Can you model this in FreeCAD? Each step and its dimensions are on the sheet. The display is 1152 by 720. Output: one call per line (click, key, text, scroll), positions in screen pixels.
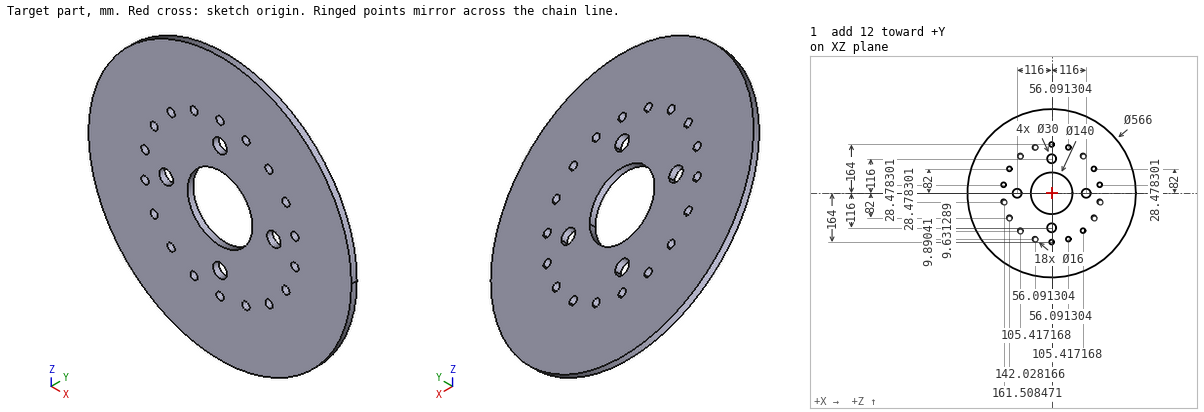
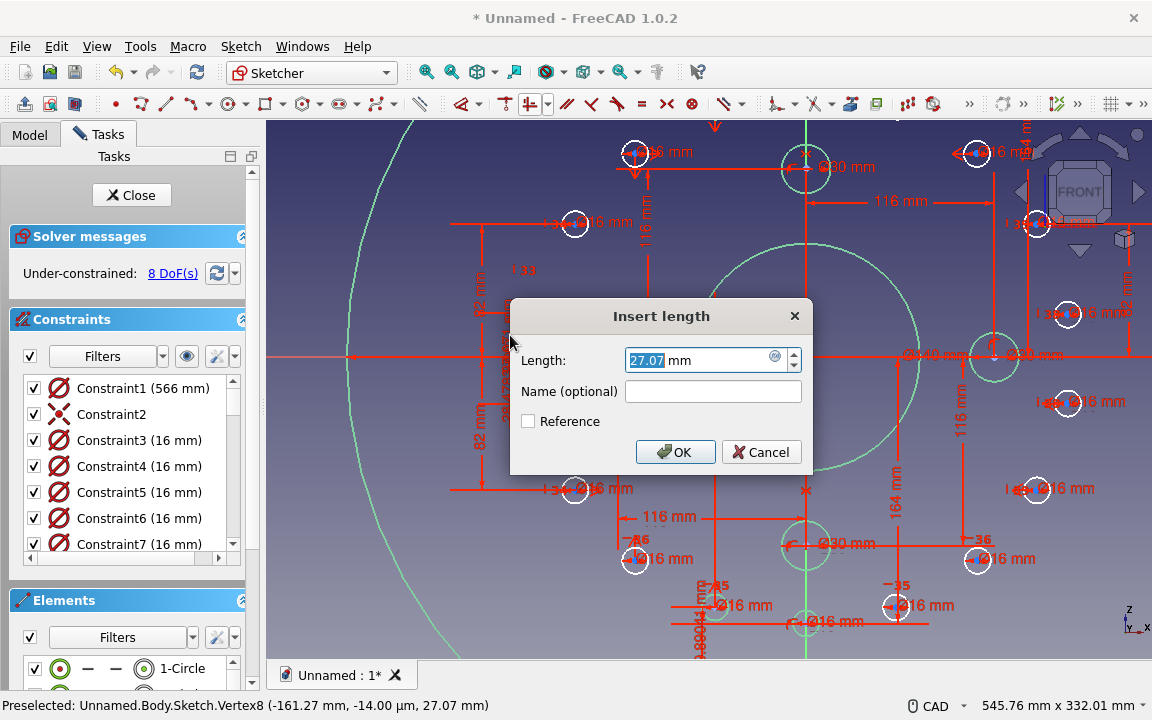
text(28.478301)
key(Return)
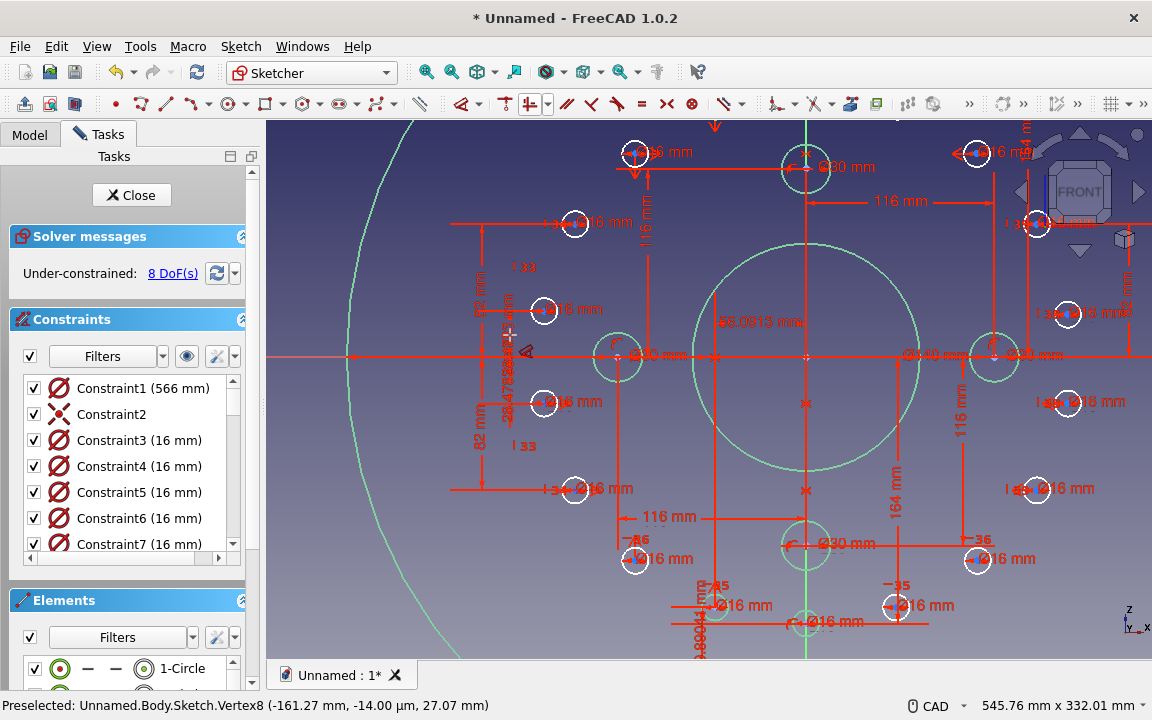
click(896, 607)
click(851, 323)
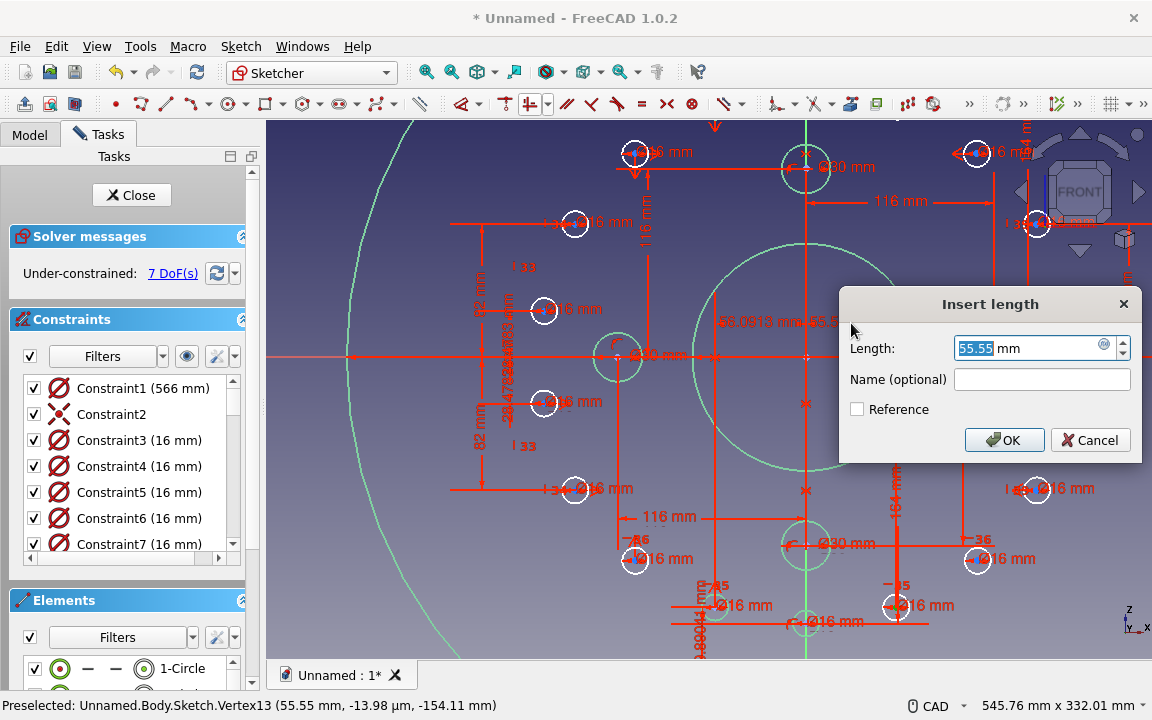
text(56.091304)
key(Return)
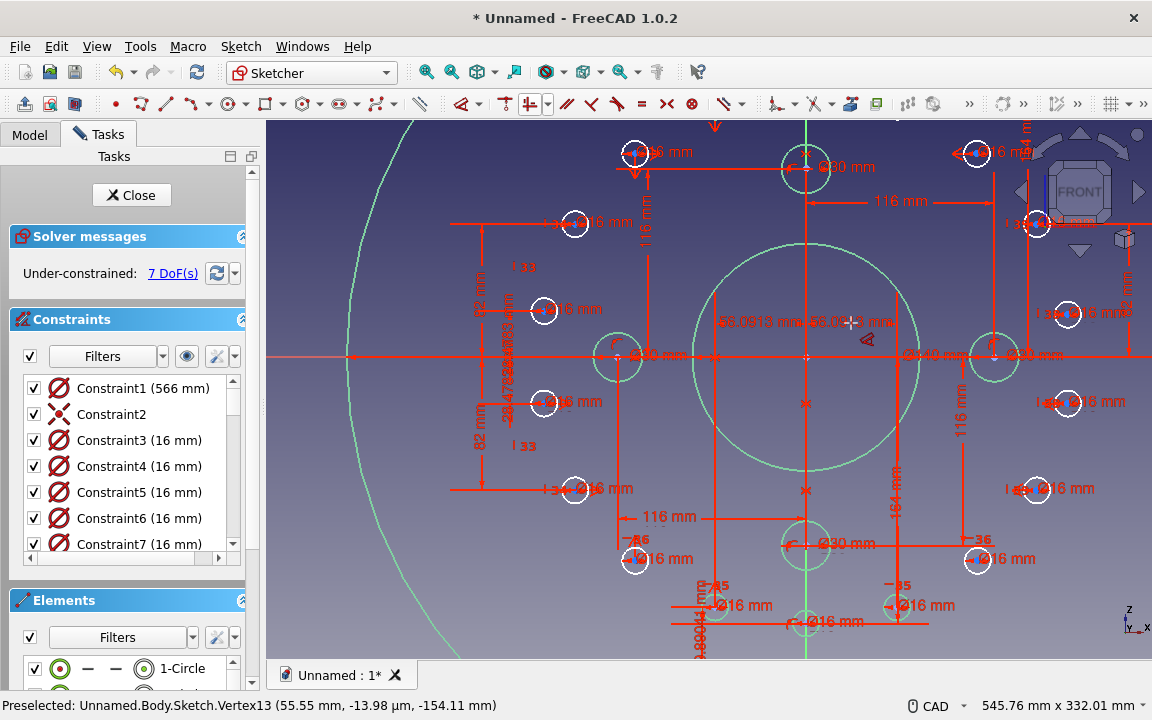
scroll(544, 408, down, 5)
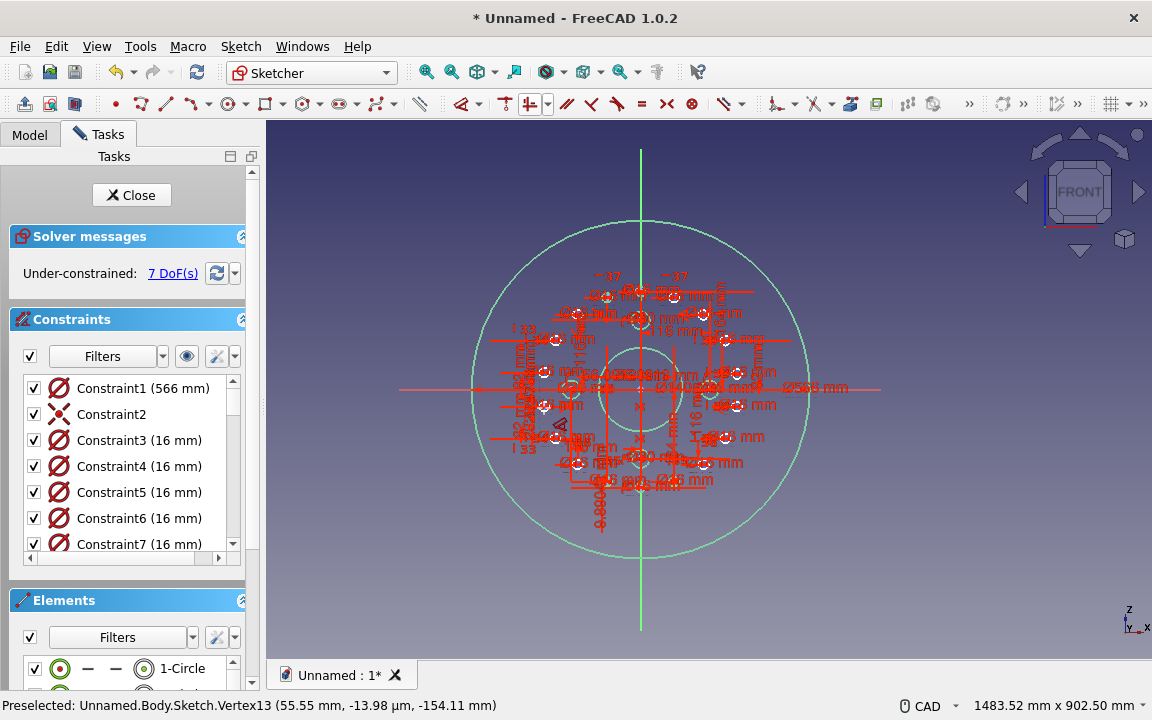
click(674, 298)
click(657, 264)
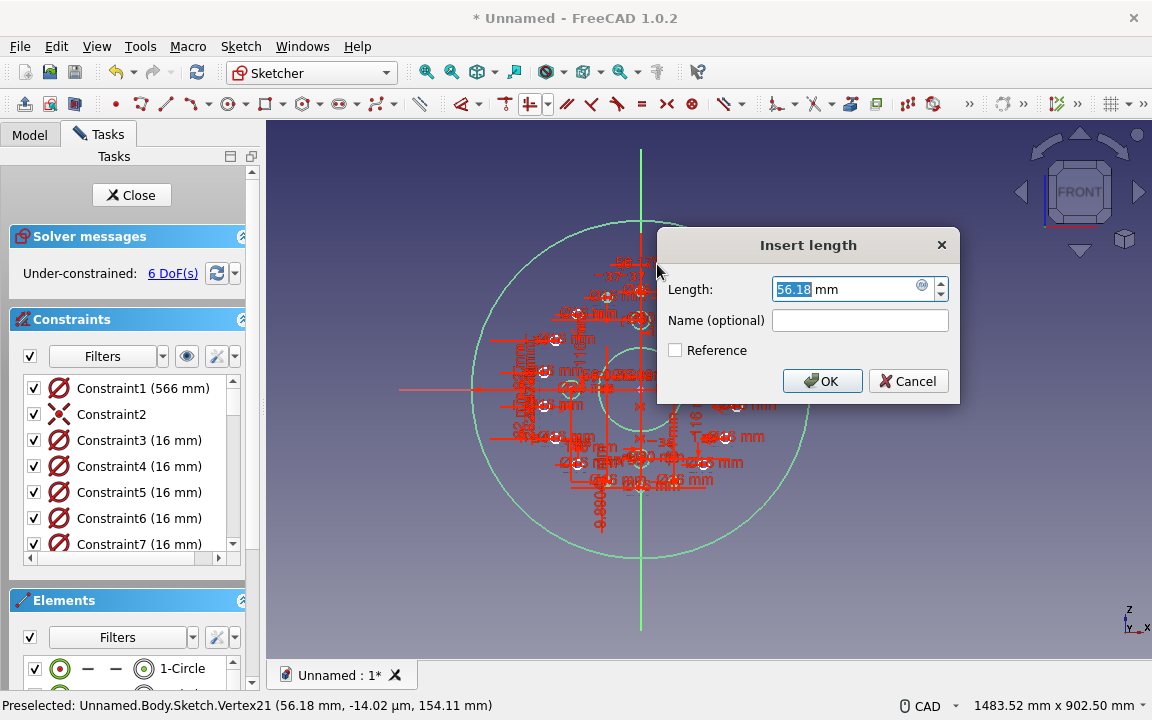
text(56.091304)
key(Return)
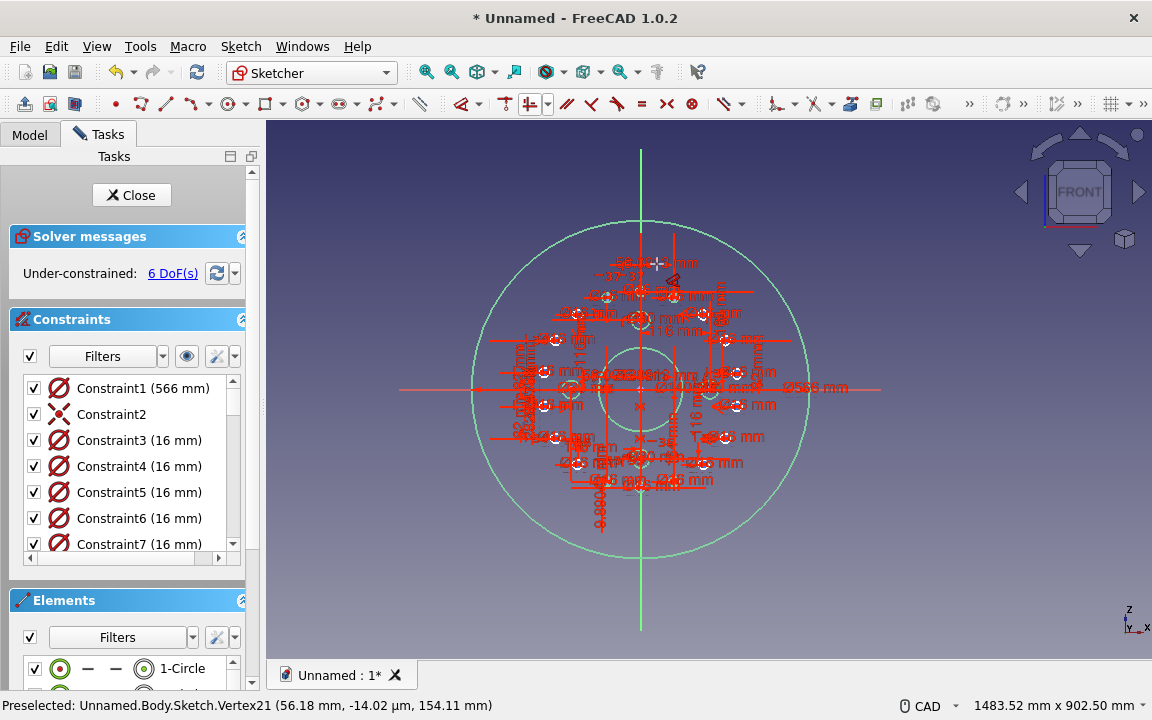
scroll(737, 374, up, 5)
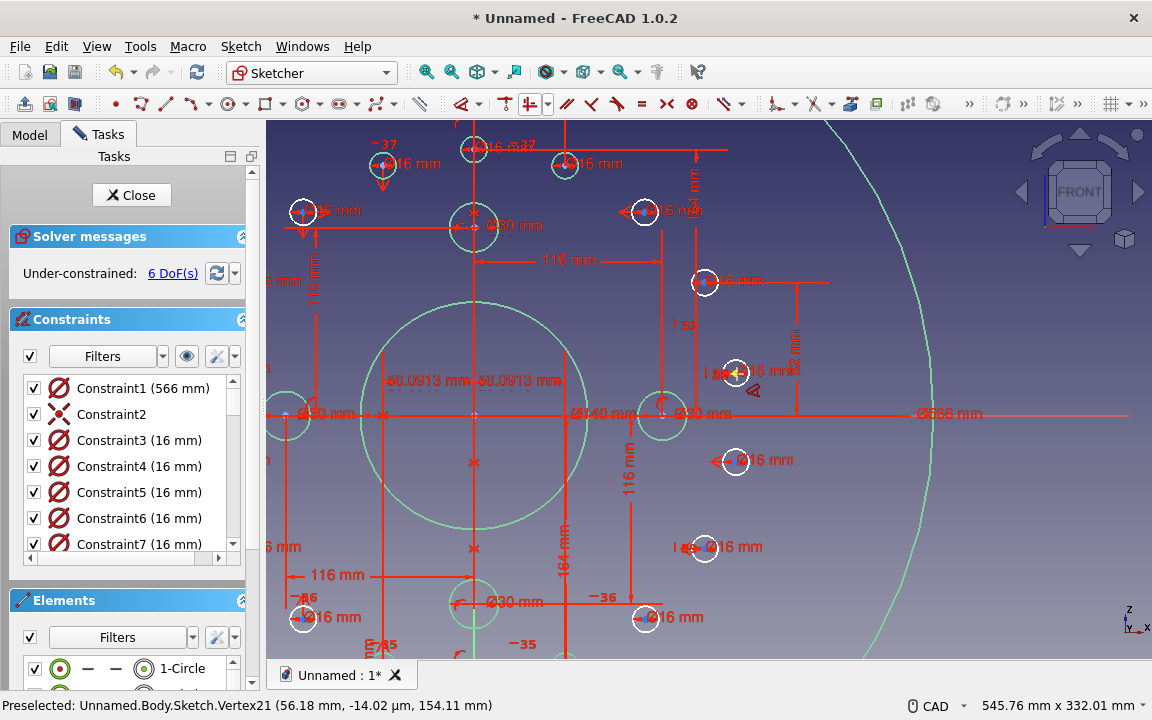
click(736, 373)
click(770, 395)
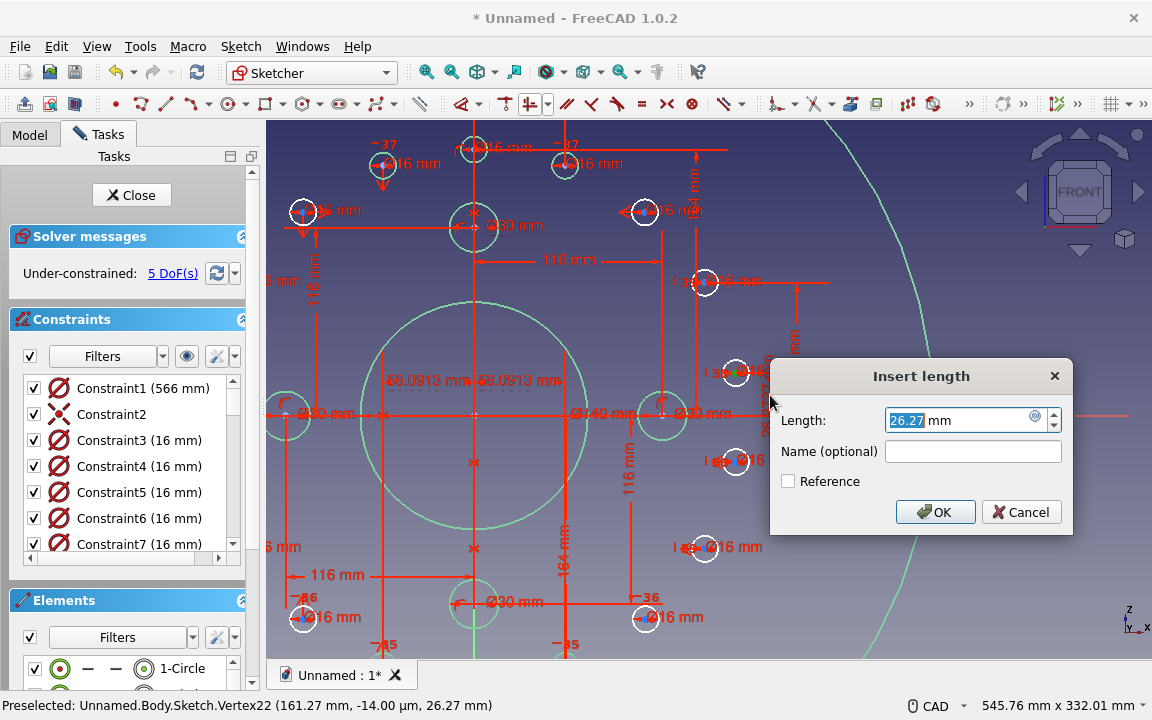
text(28.478301)
key(Return)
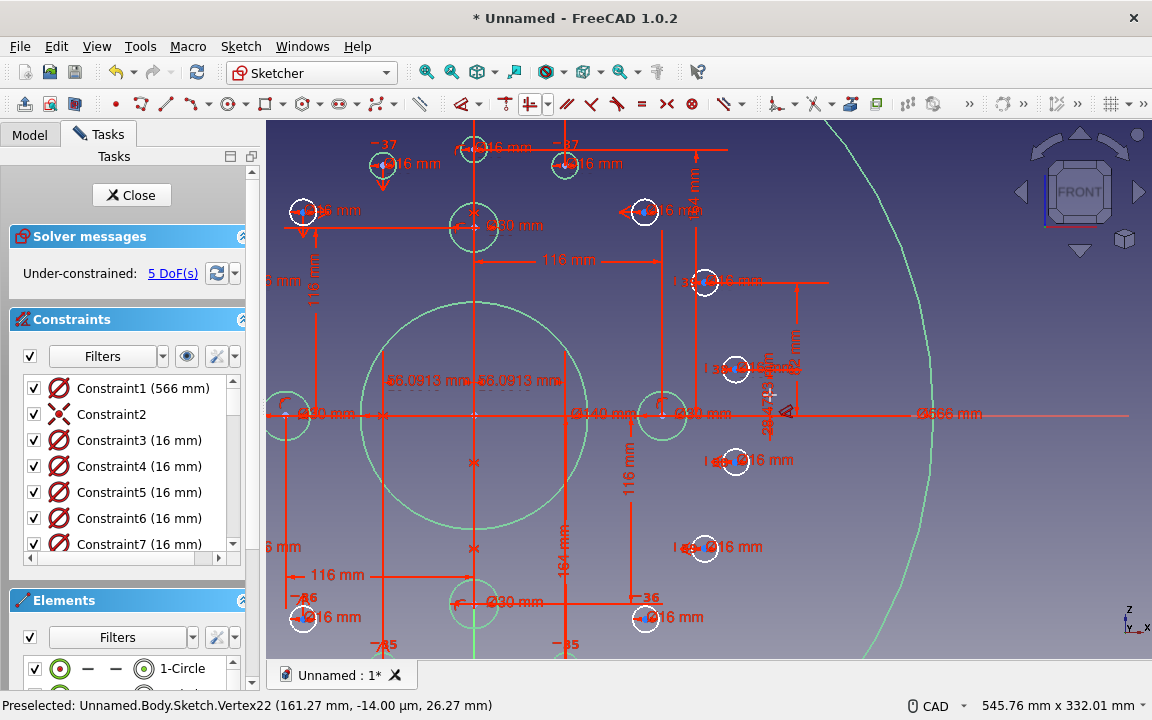
scroll(303, 619, up, 5)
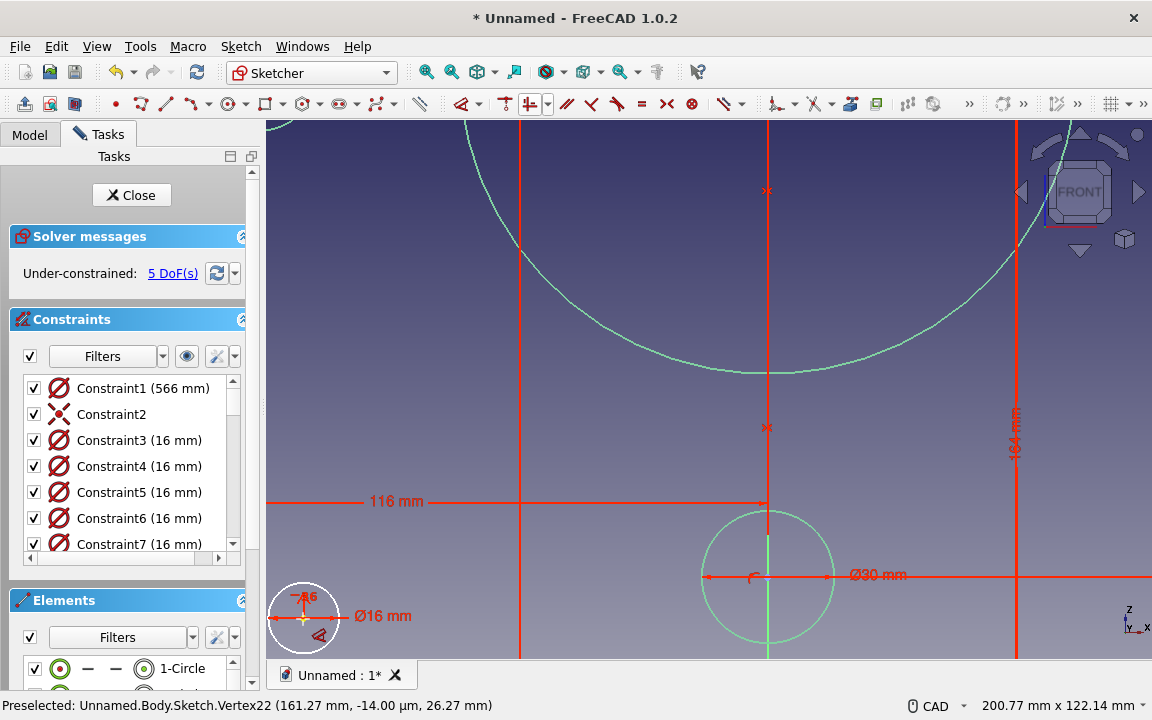
click(304, 618)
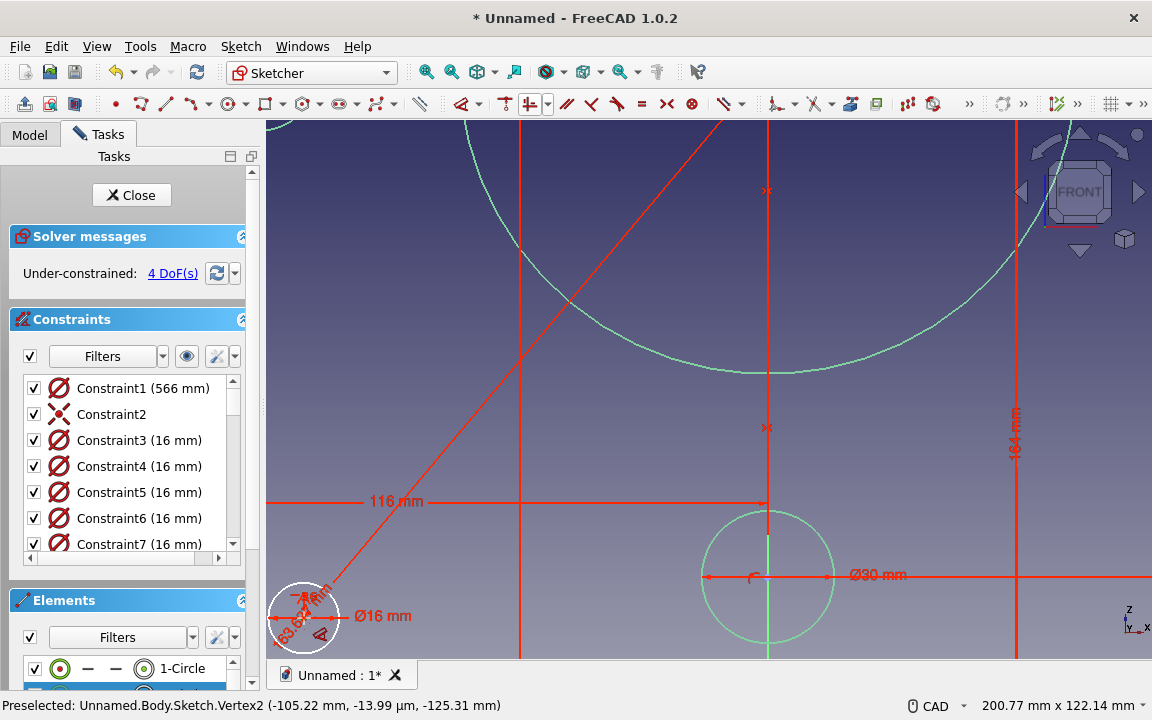
click(768, 577)
click(802, 598)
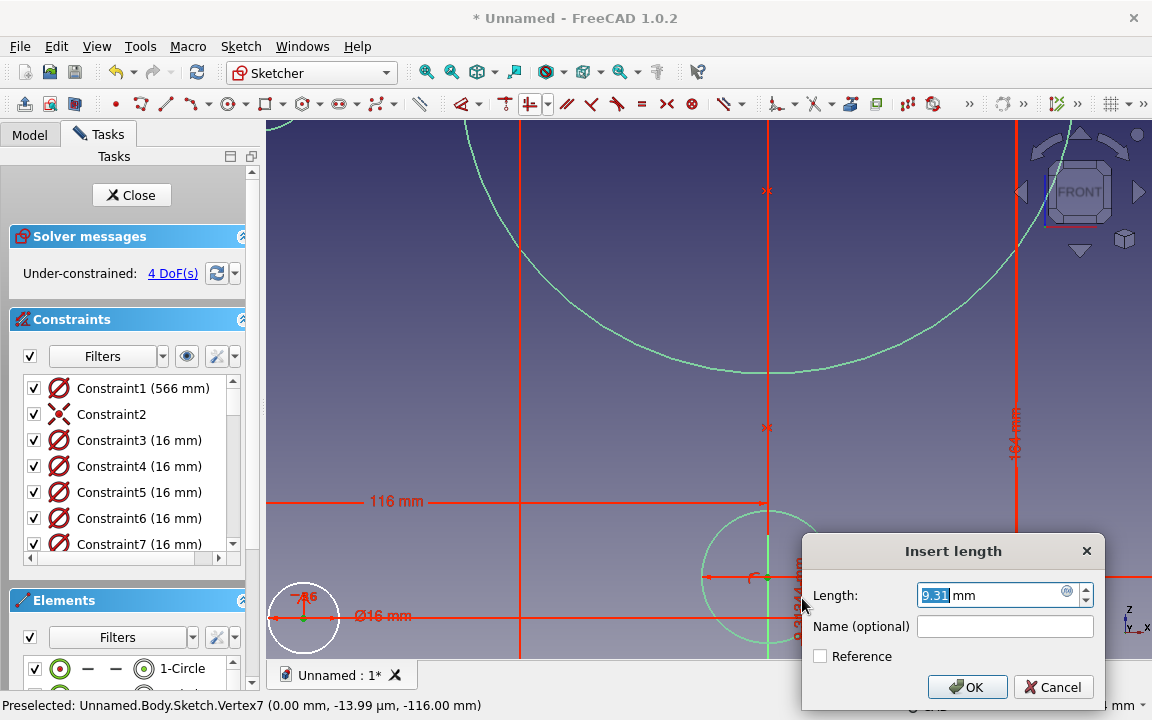
text(9.631289)
key(Return)